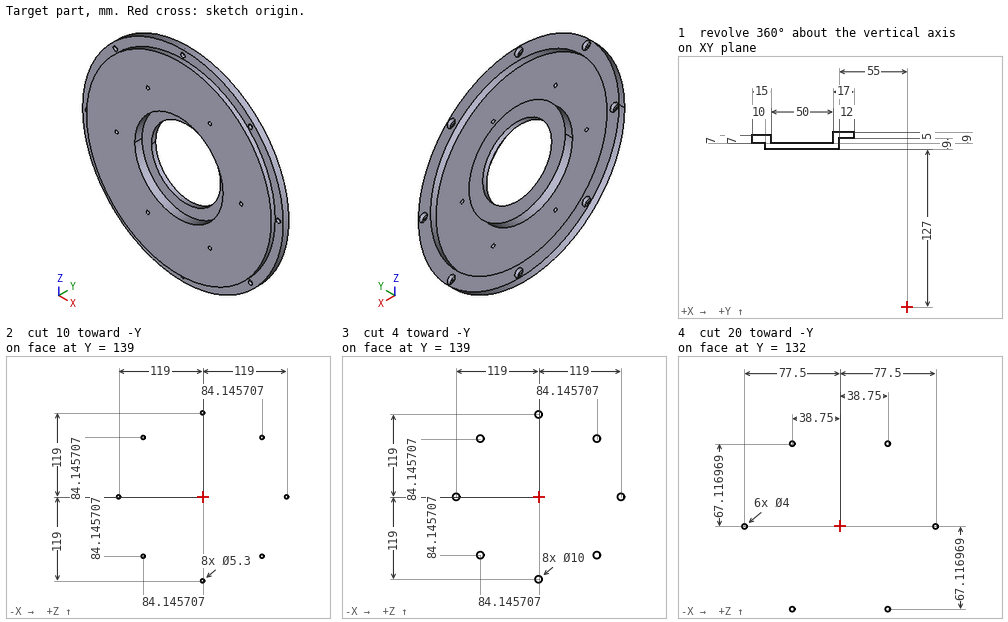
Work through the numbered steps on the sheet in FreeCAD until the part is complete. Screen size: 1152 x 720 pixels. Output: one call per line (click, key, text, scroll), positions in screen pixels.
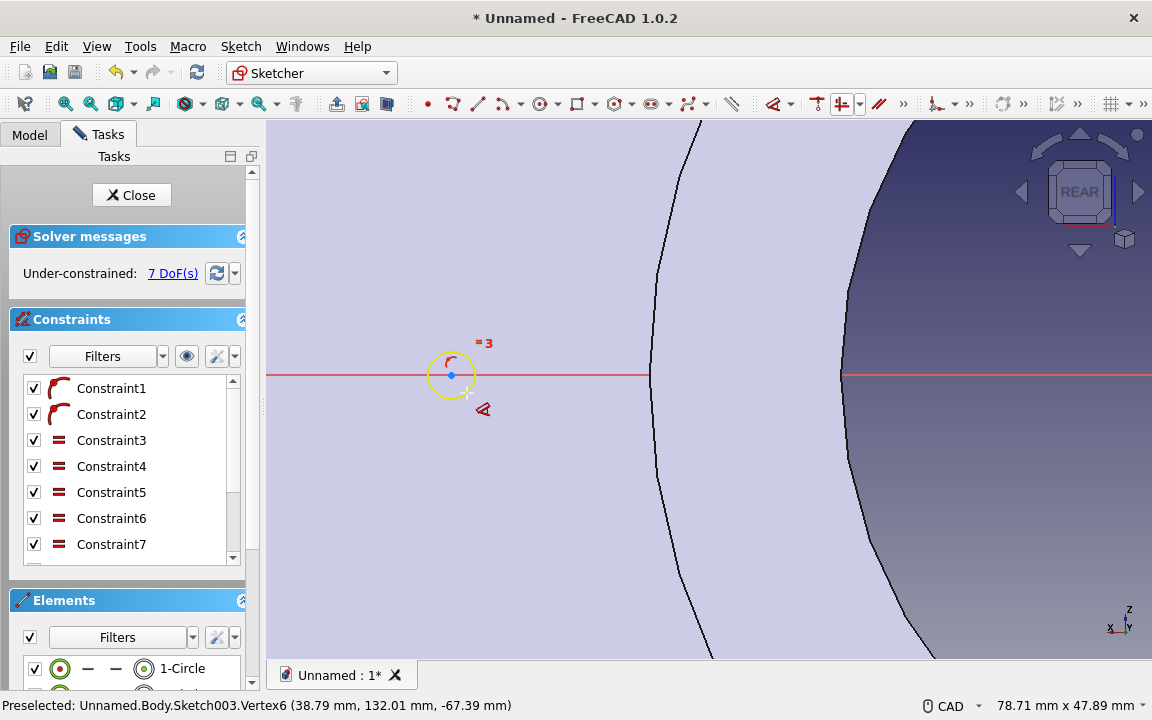
click(468, 392)
click(490, 415)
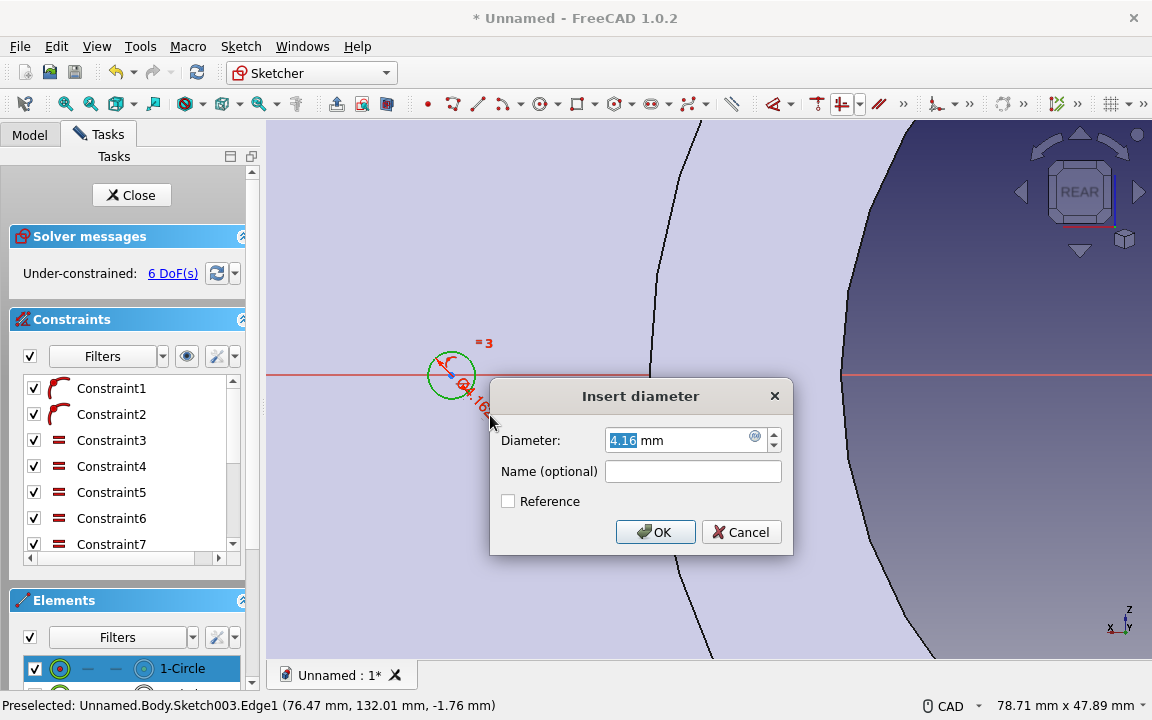
text(4)
key(Return)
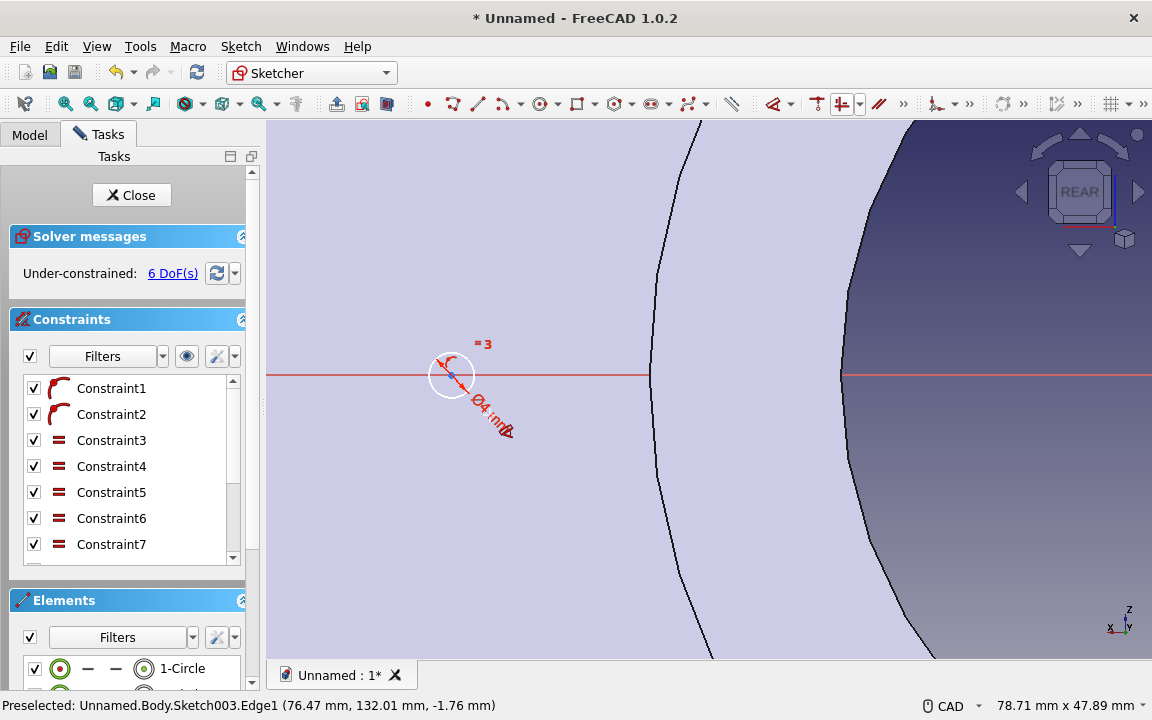
scroll(467, 393, down, 8)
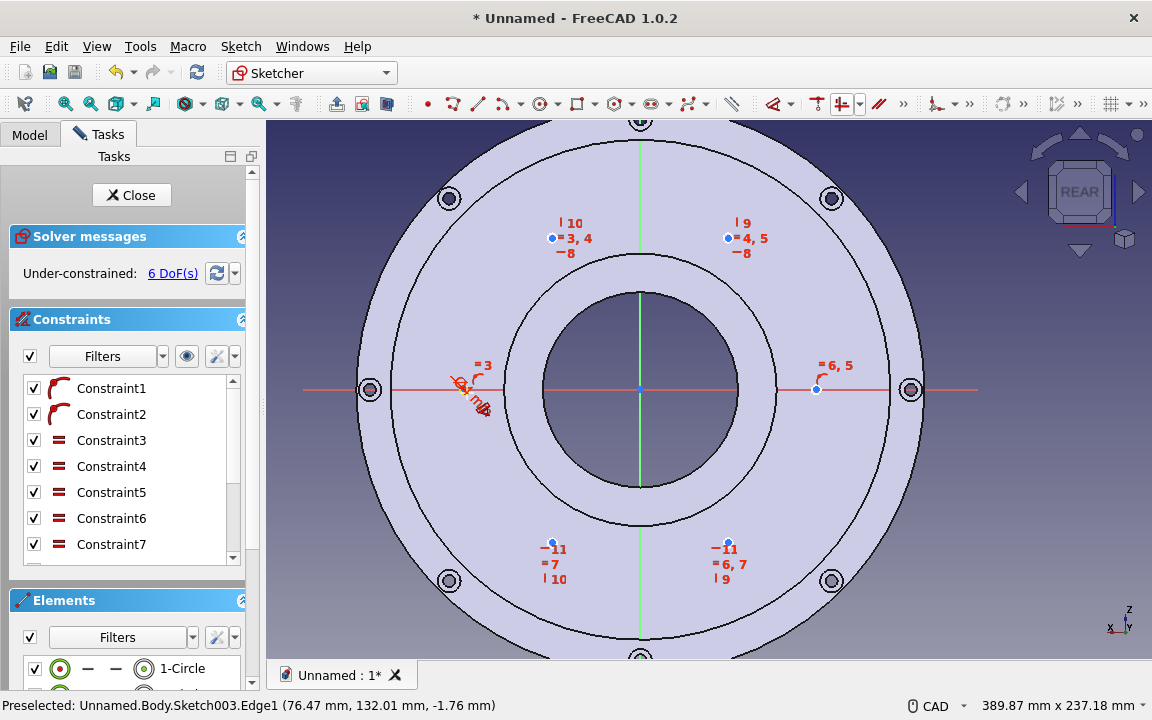
click(464, 390)
click(552, 424)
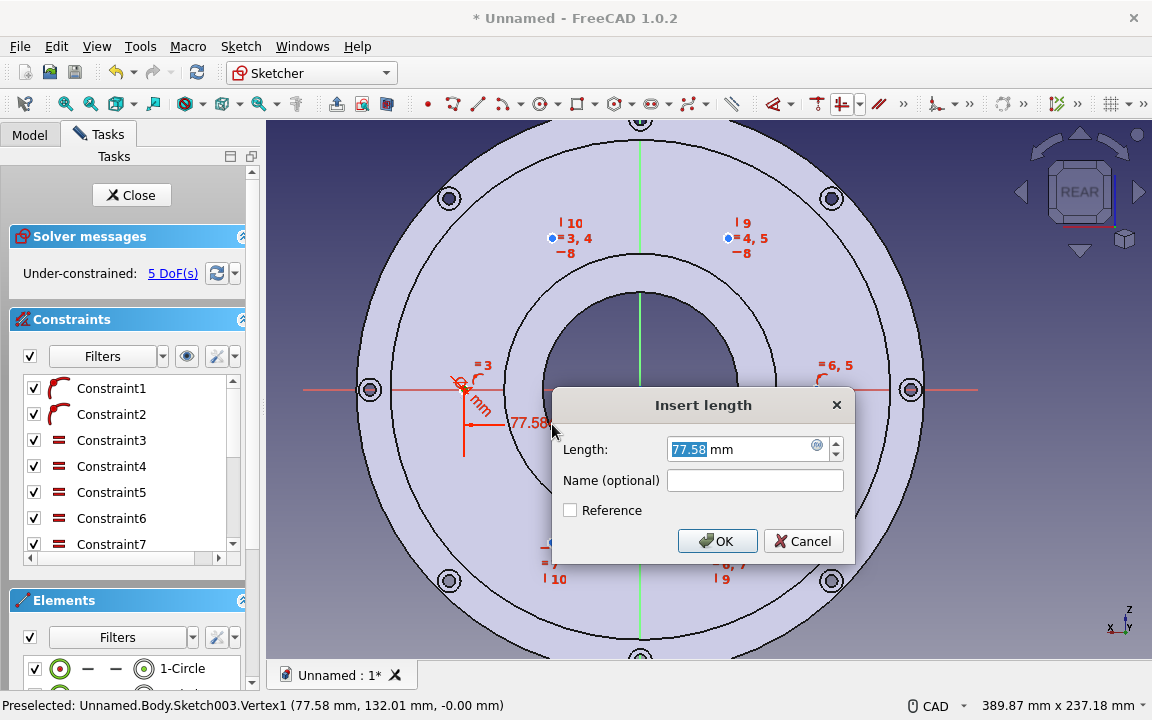
text(77.5)
key(Return)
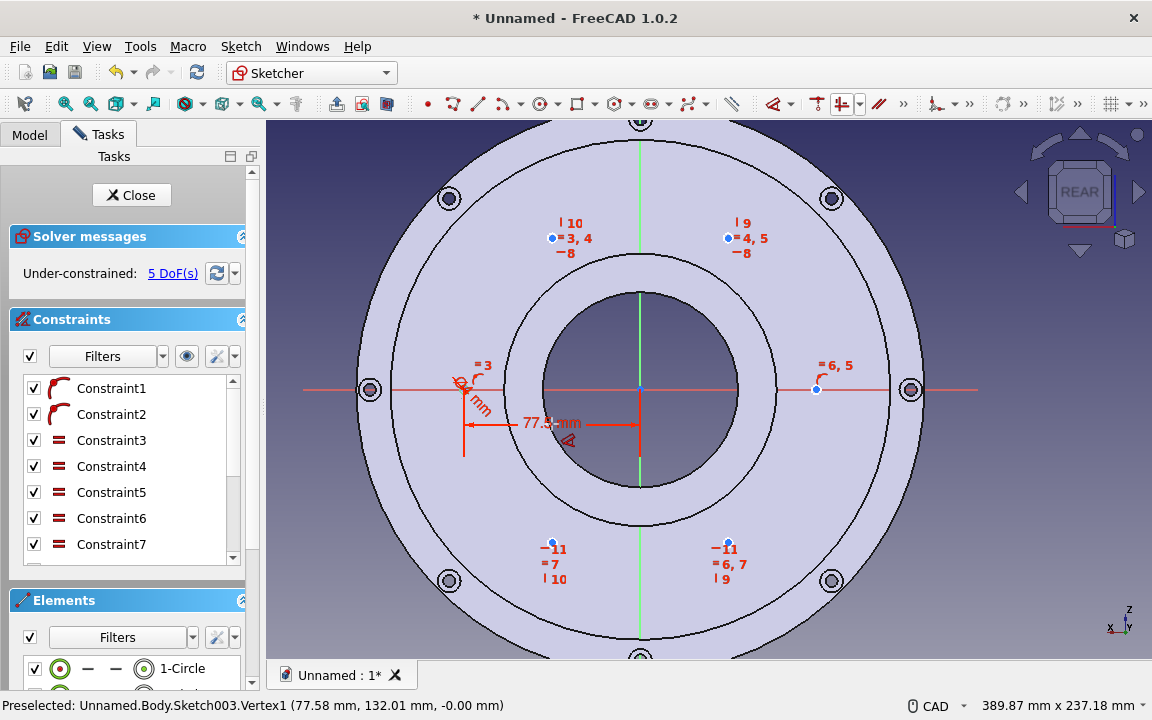
click(816, 390)
click(728, 424)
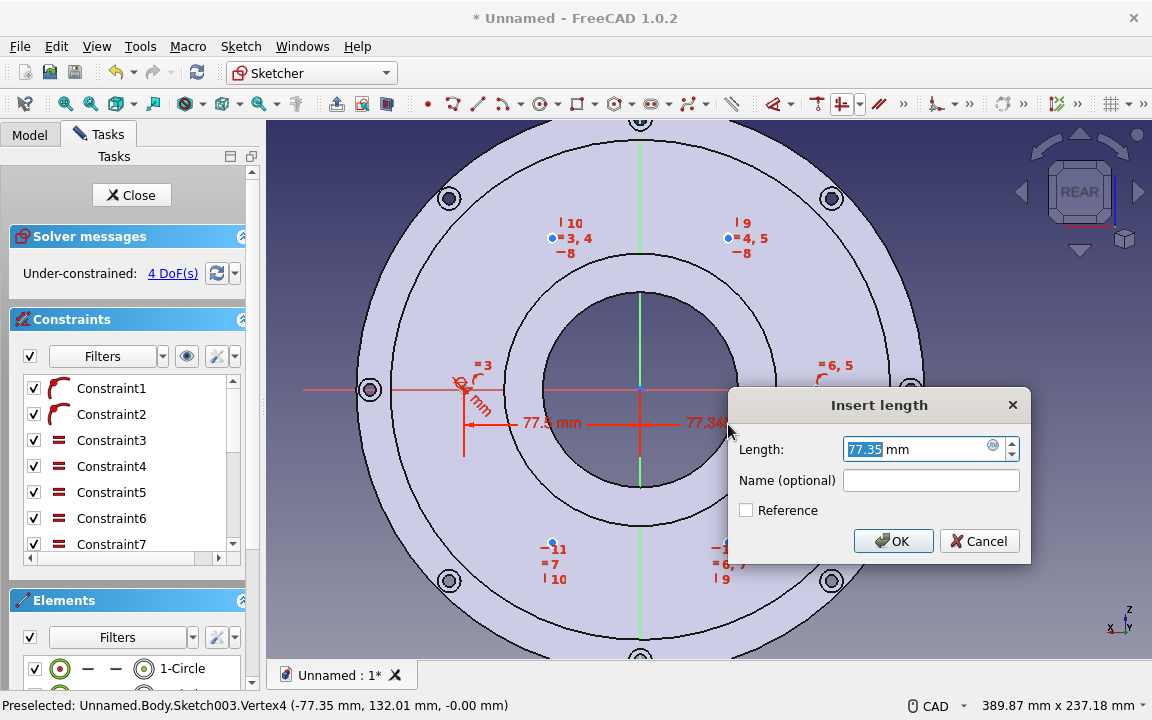
text(77.5)
key(Return)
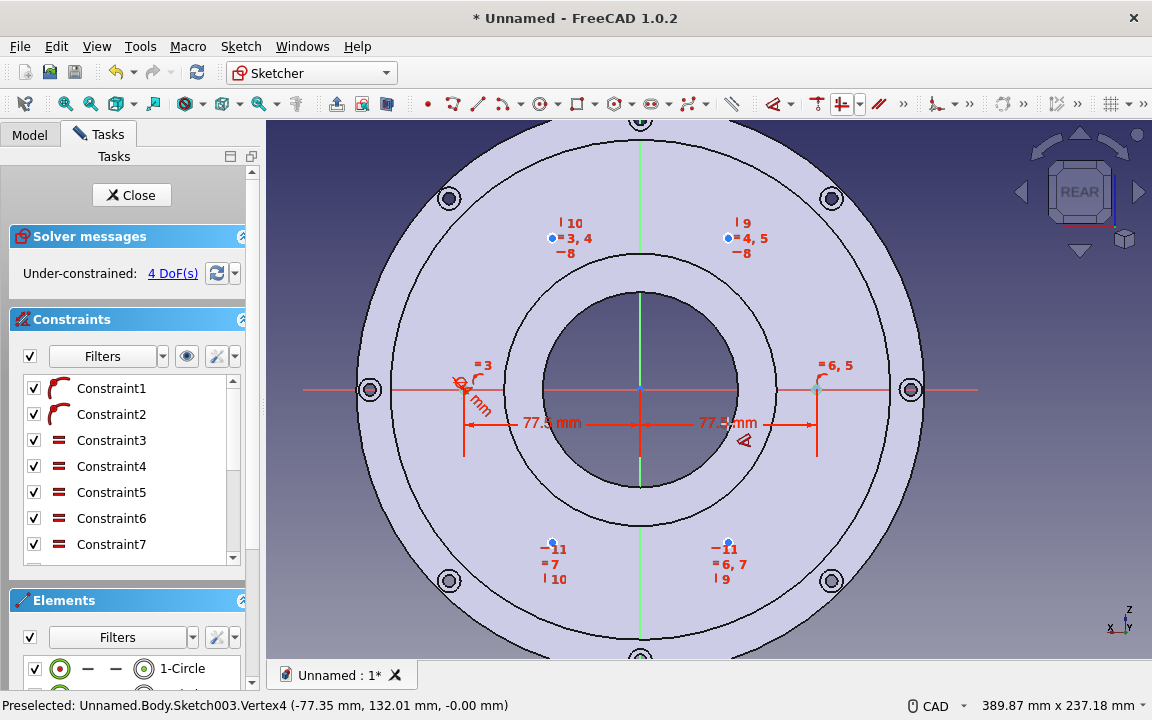
click(552, 238)
click(596, 204)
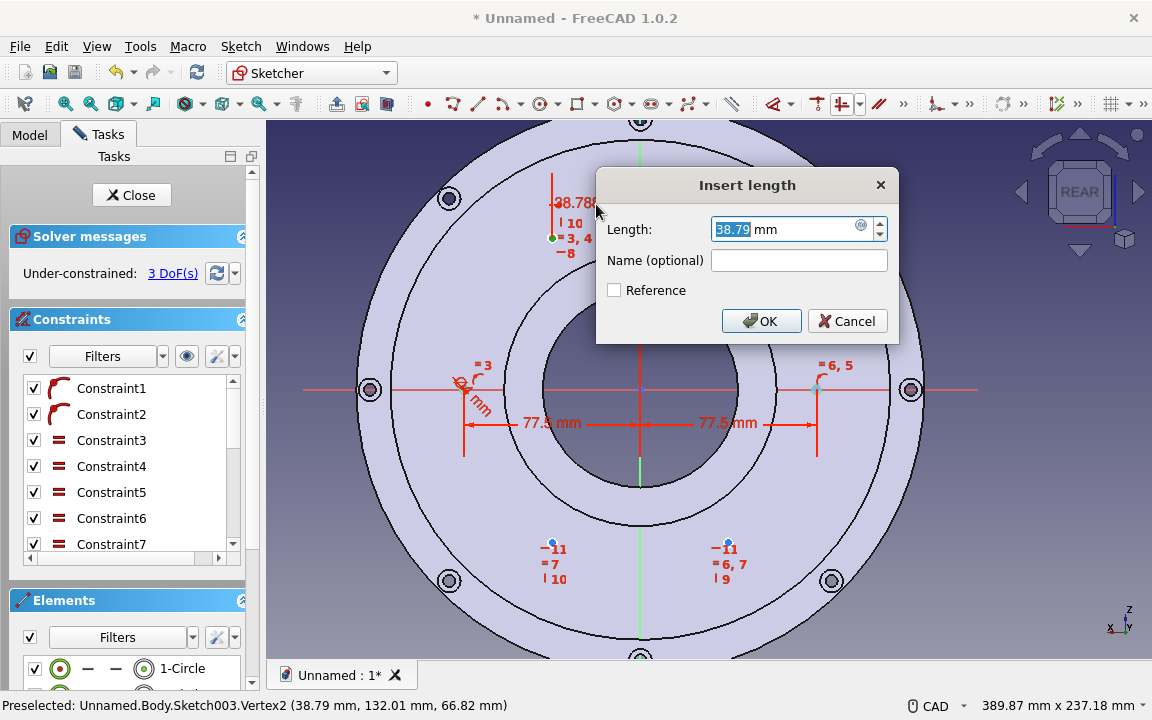
text(38.75)
key(Return)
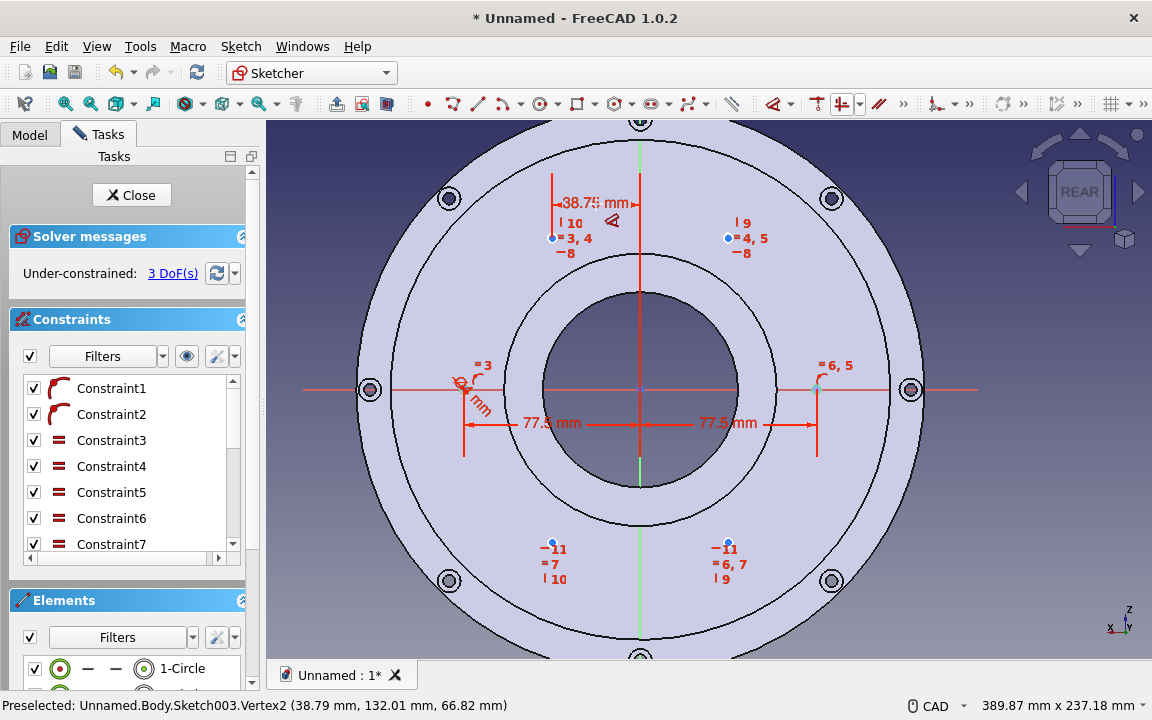
click(728, 238)
click(684, 204)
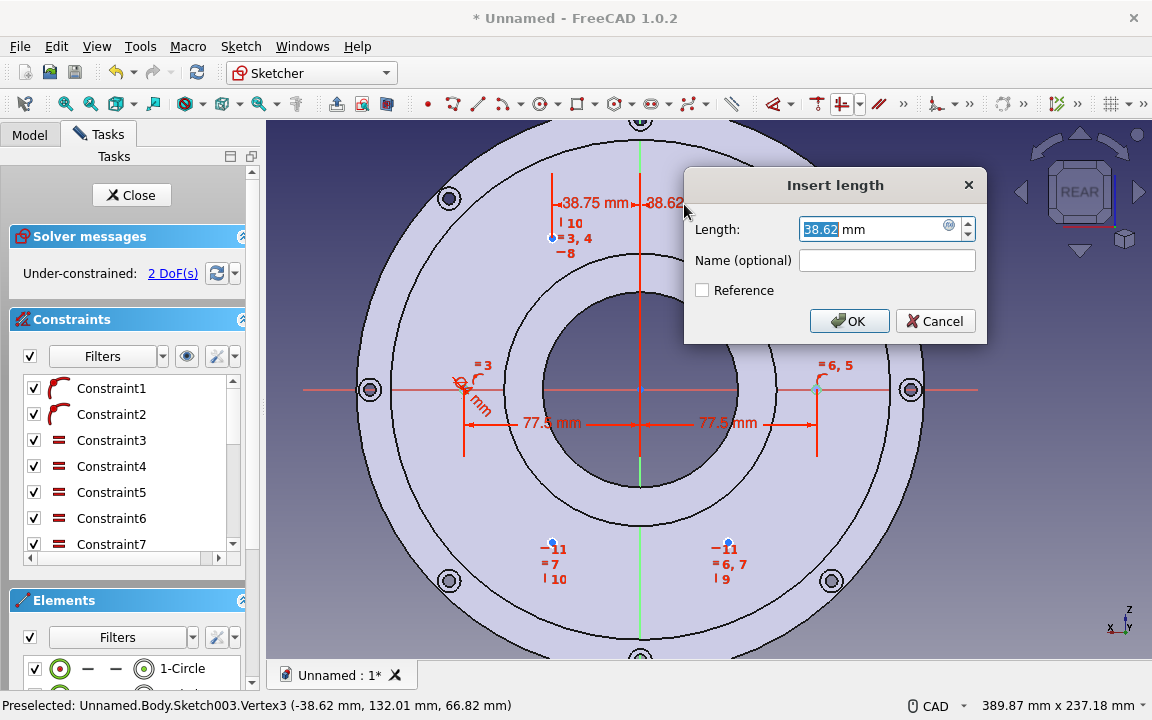
text(38.75)
key(Return)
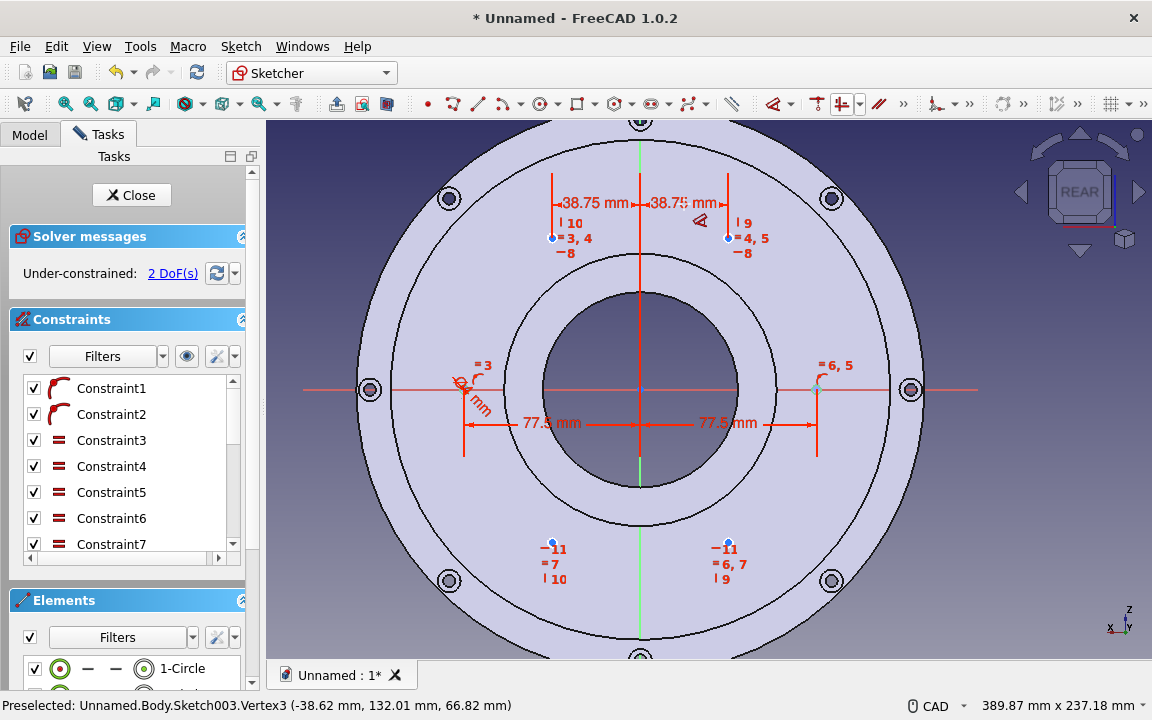
click(552, 238)
click(518, 314)